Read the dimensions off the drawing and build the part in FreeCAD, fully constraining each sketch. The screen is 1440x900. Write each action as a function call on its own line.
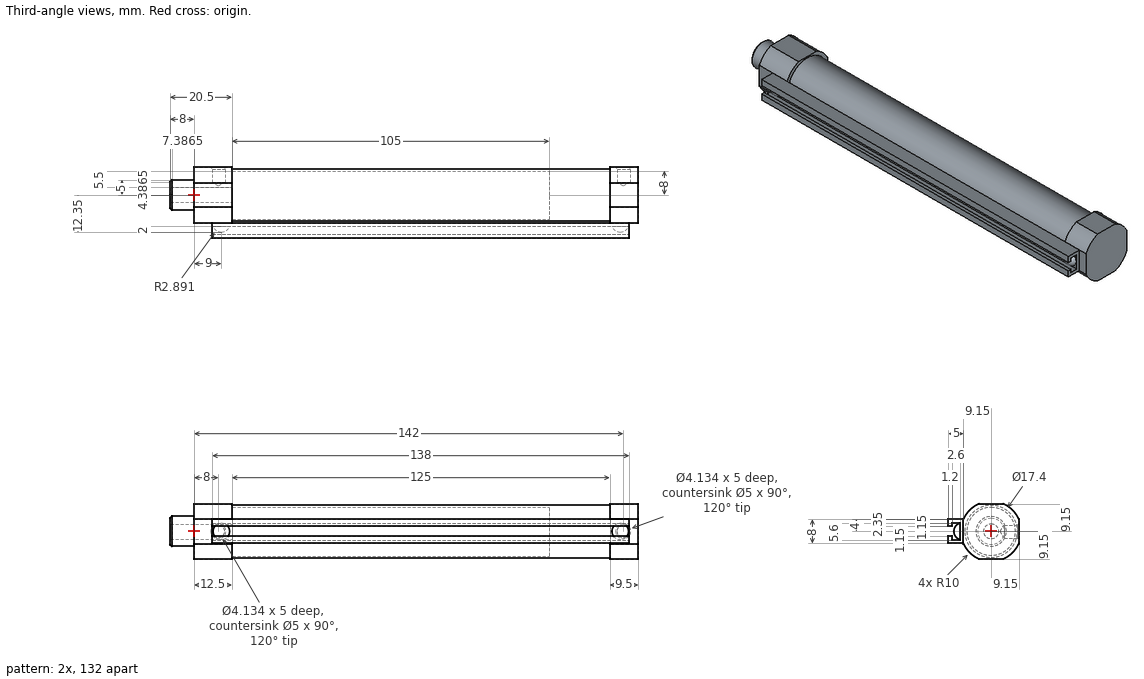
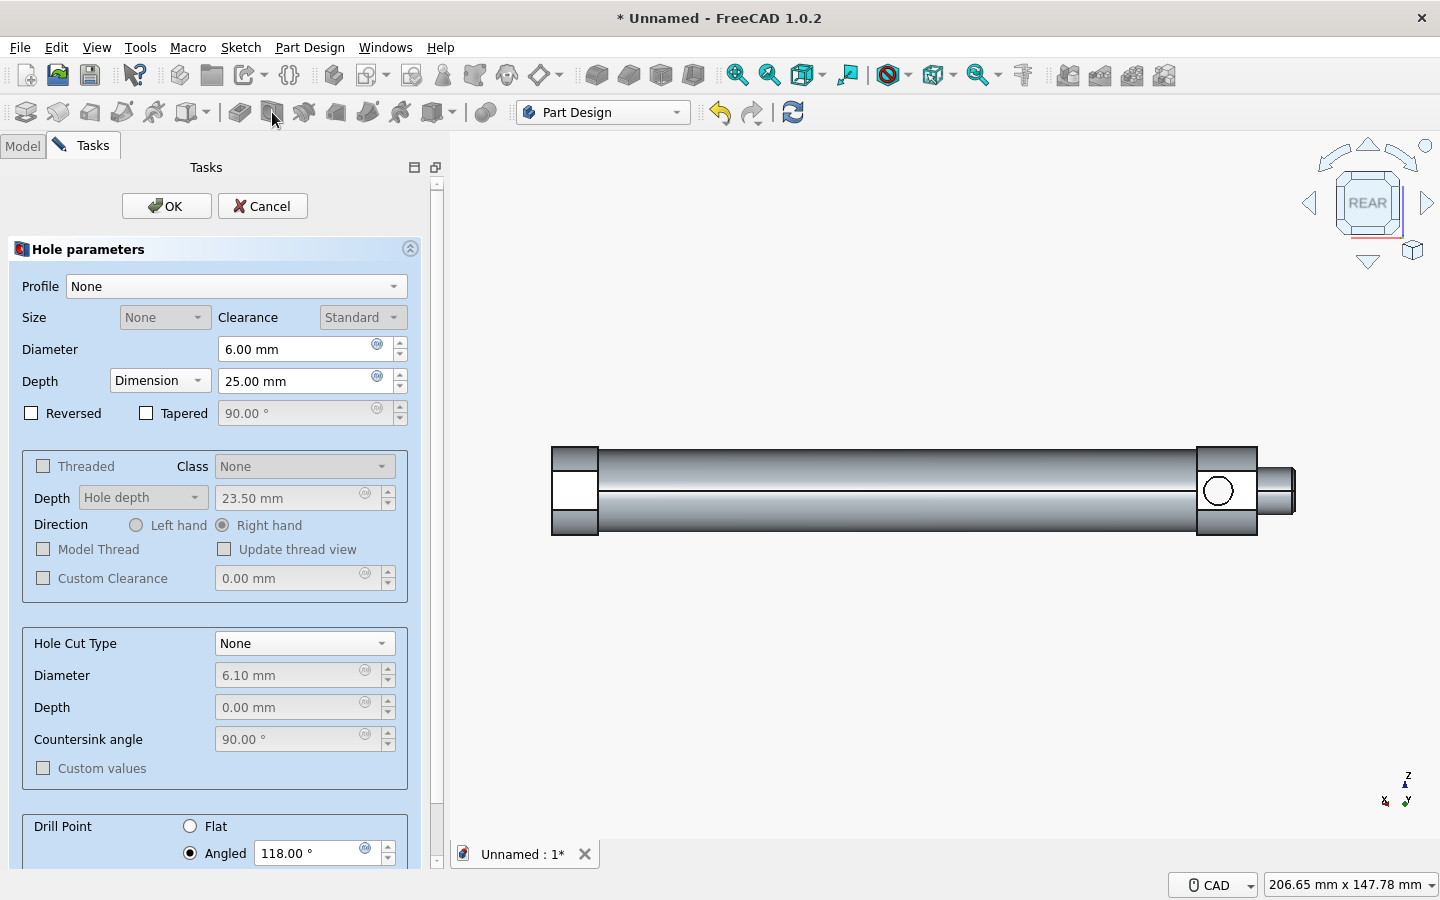
triple_click(305, 349)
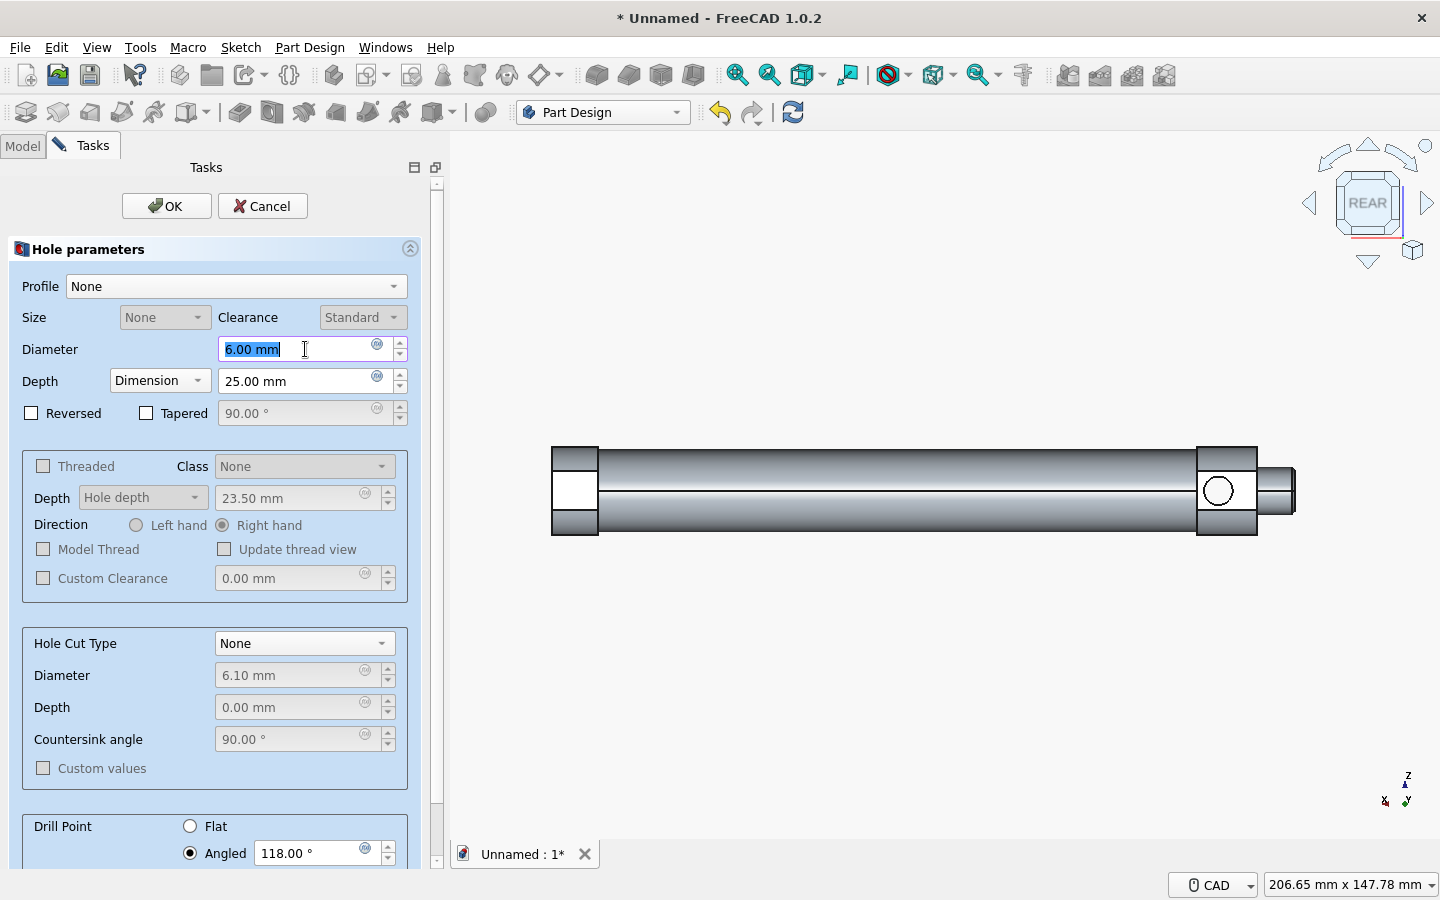
text(4.134)
key(Tab)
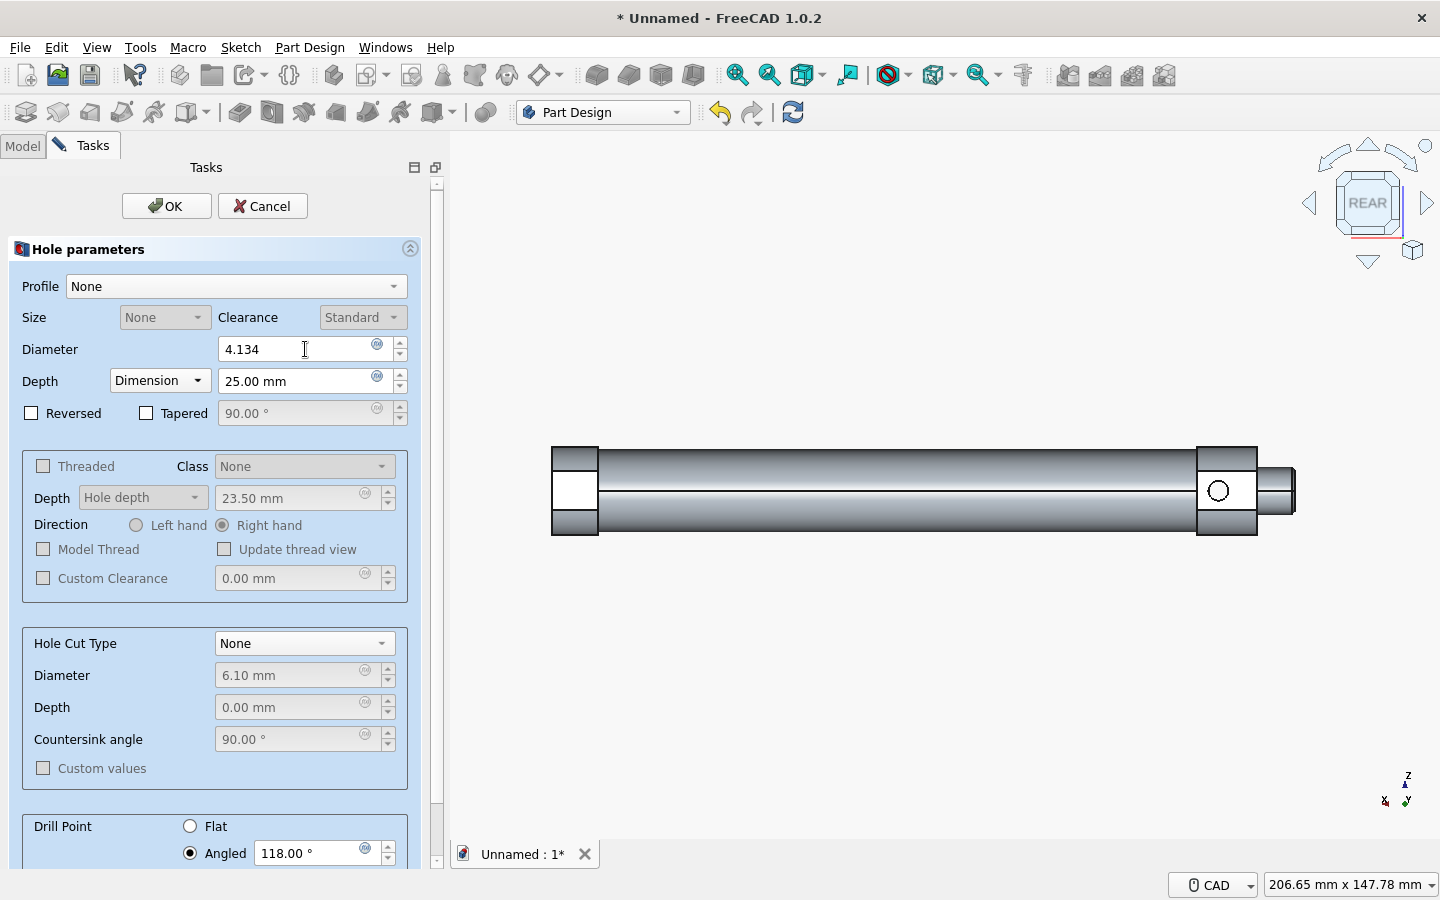
triple_click(305, 381)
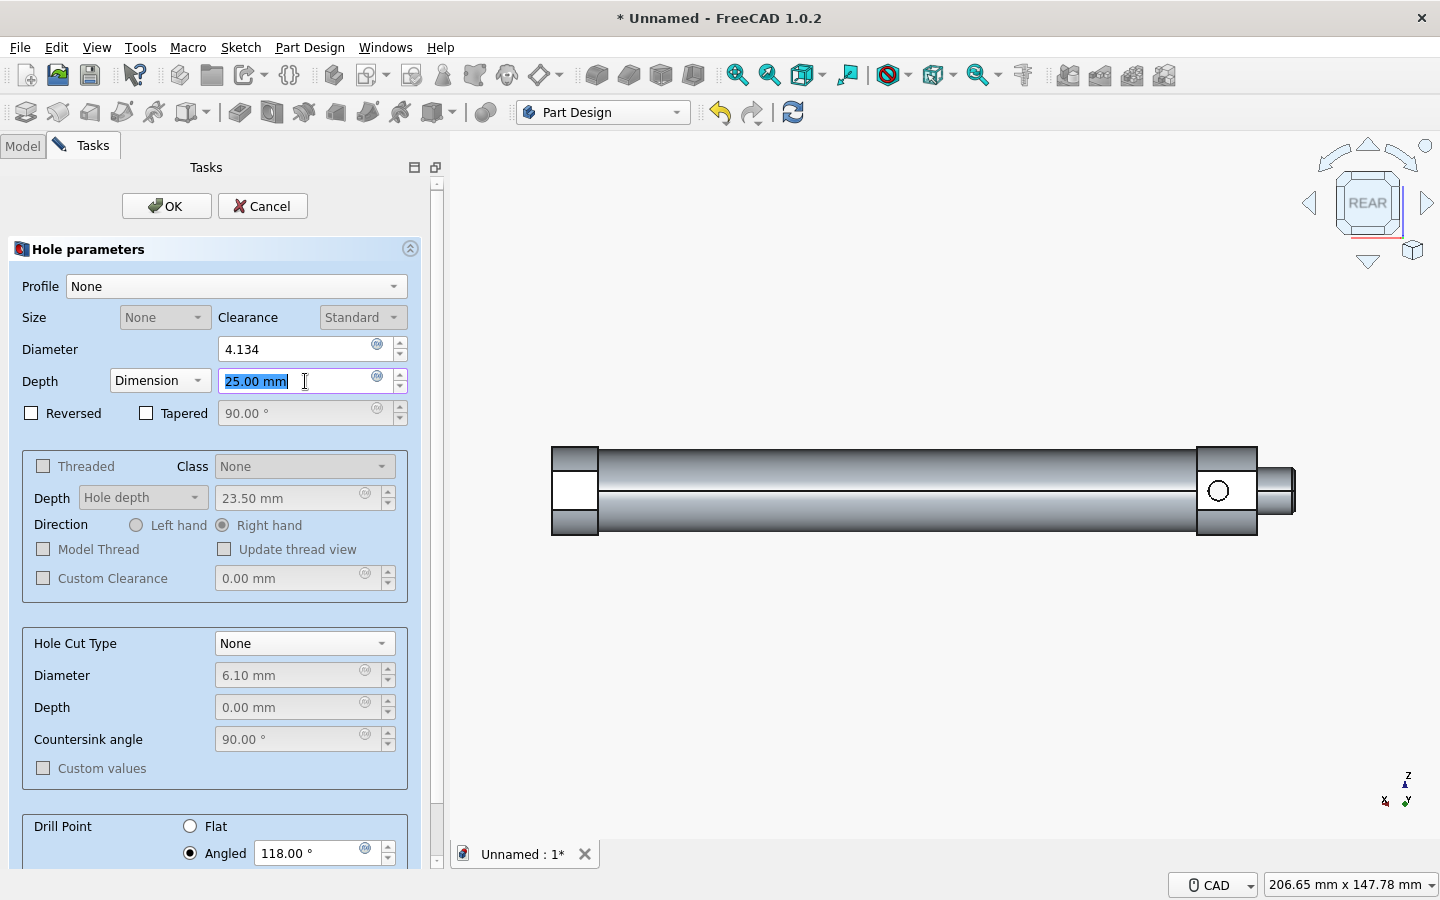
text(5)
key(Tab)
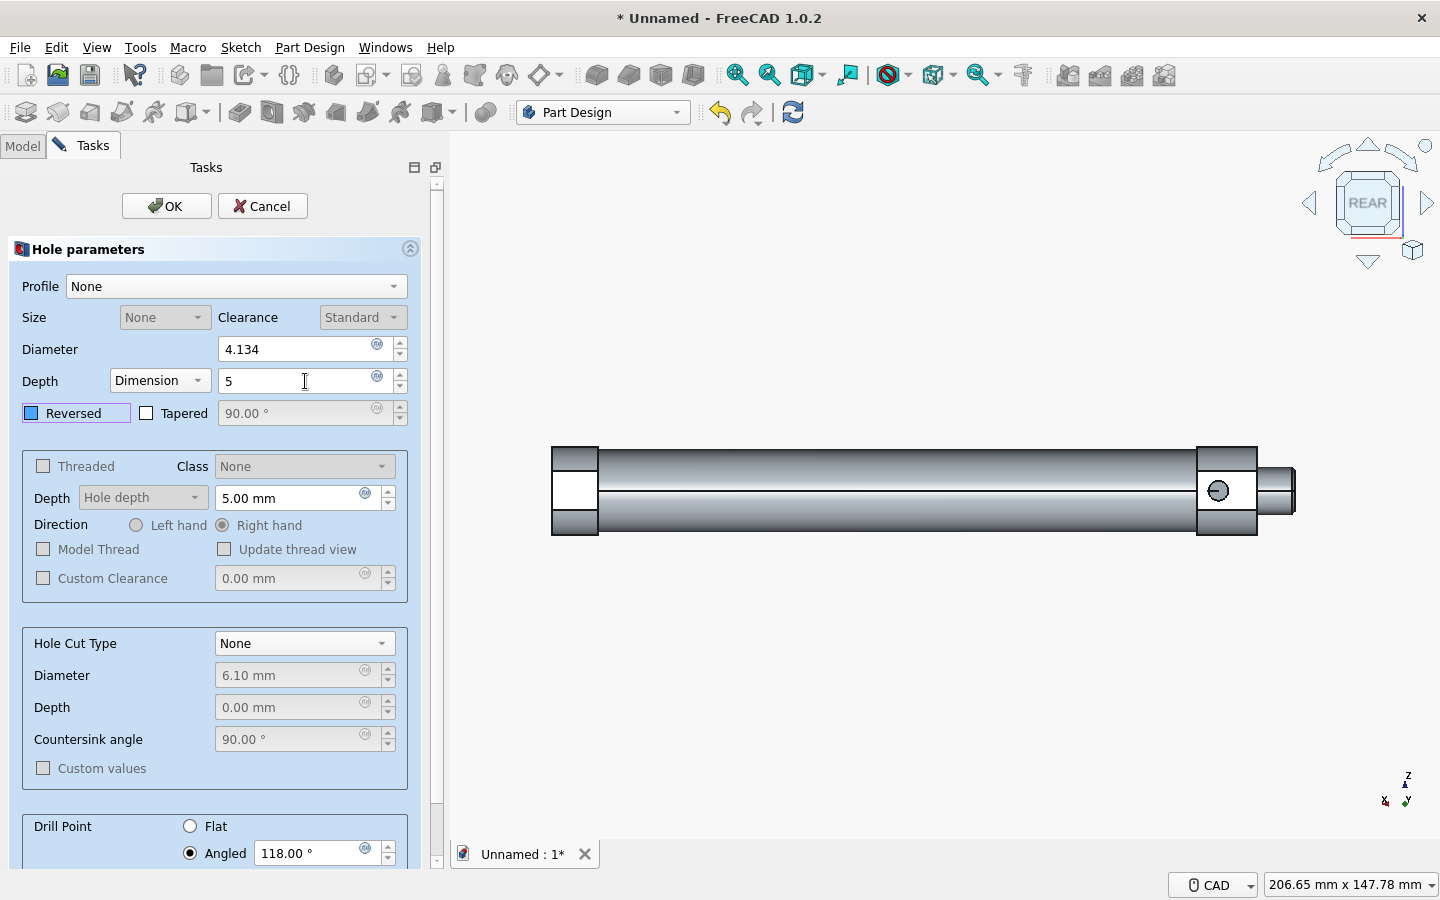
click(306, 644)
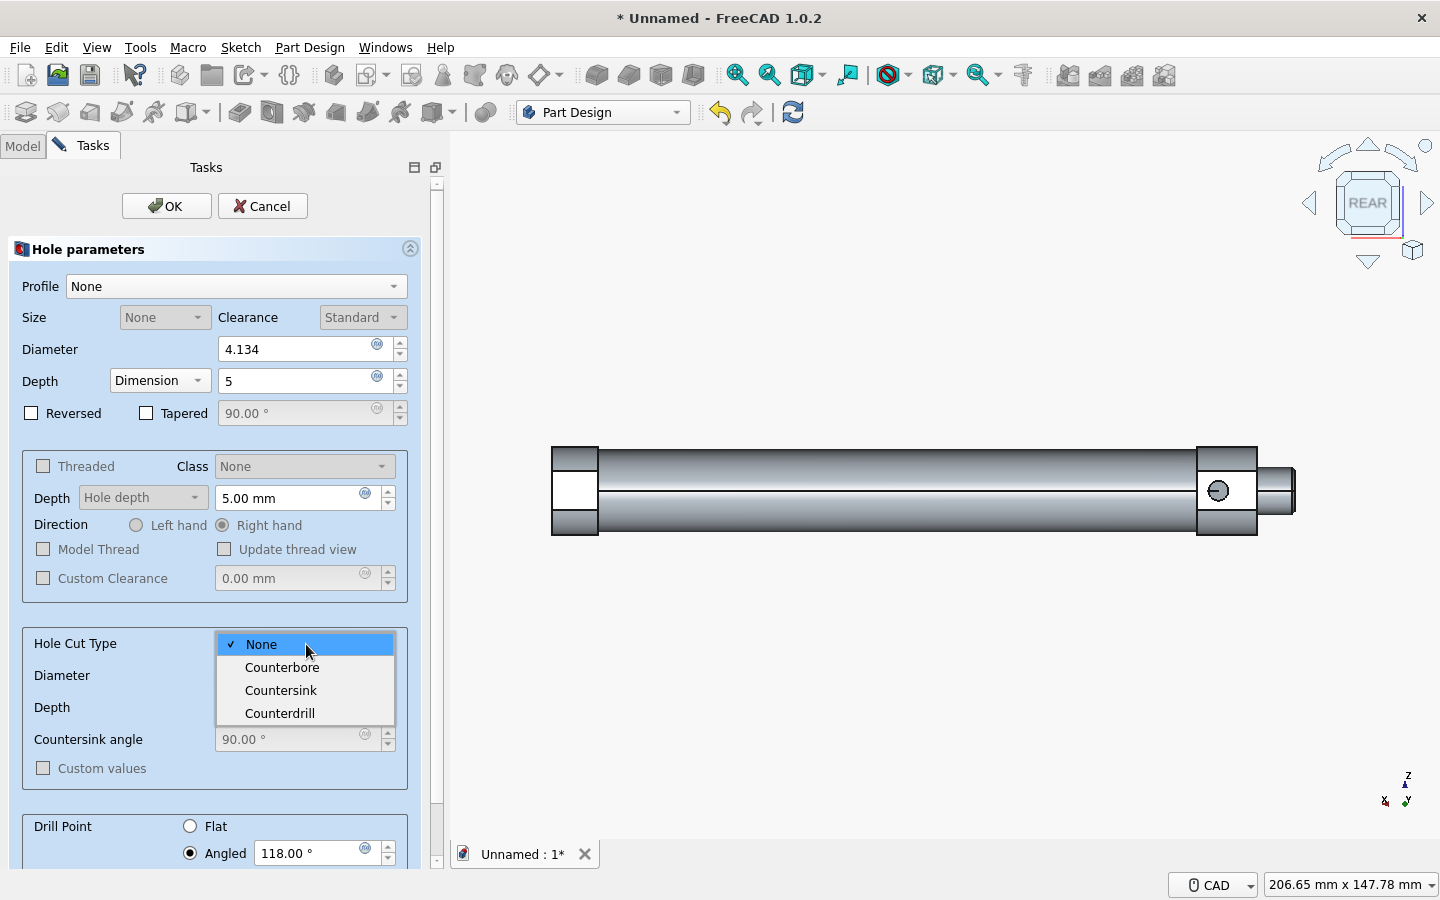
click(304, 690)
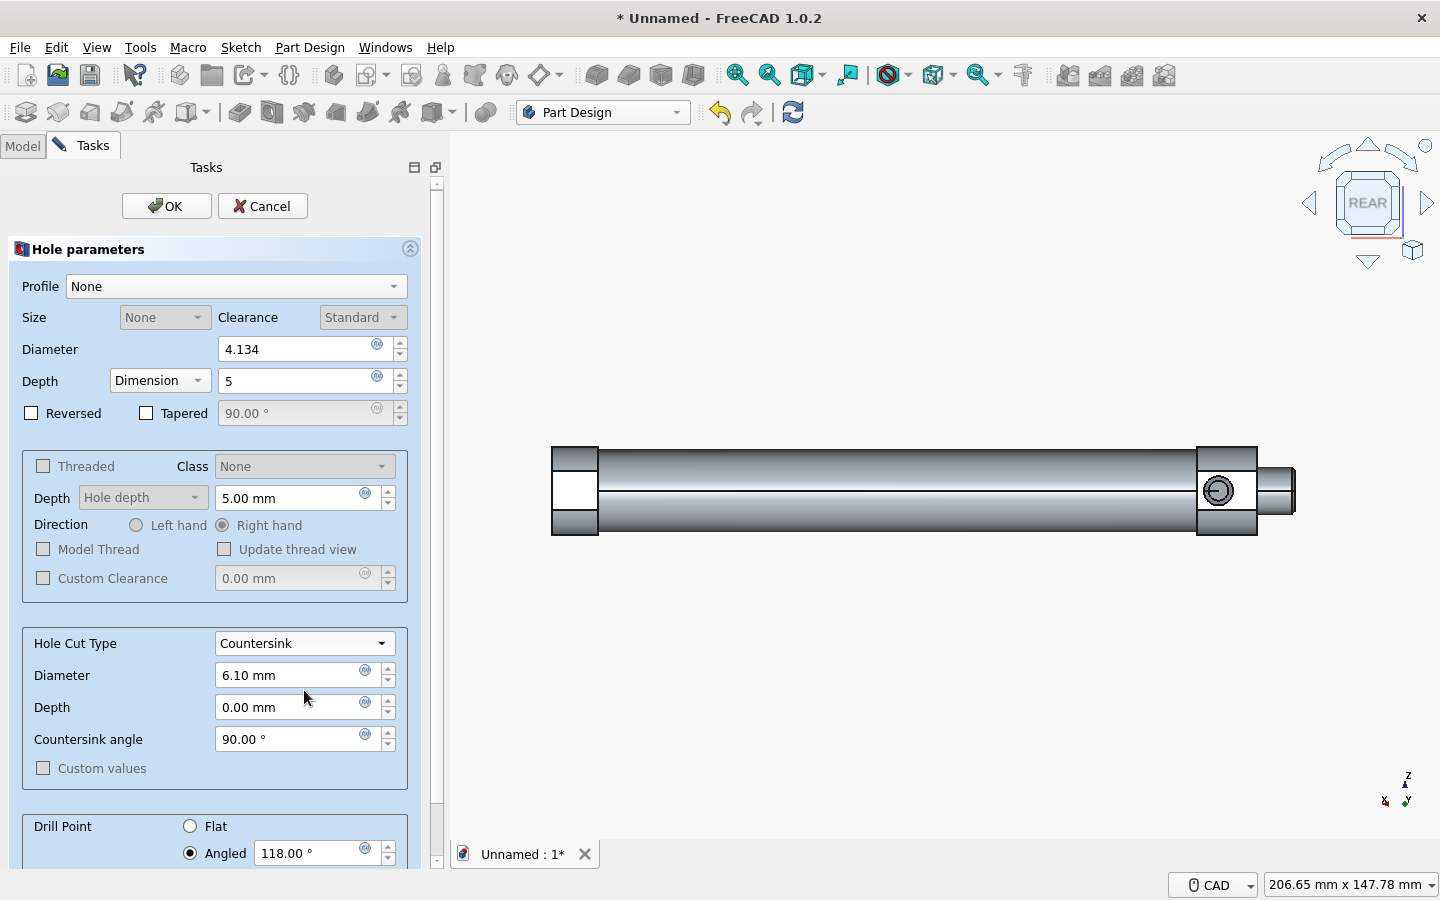
triple_click(298, 675)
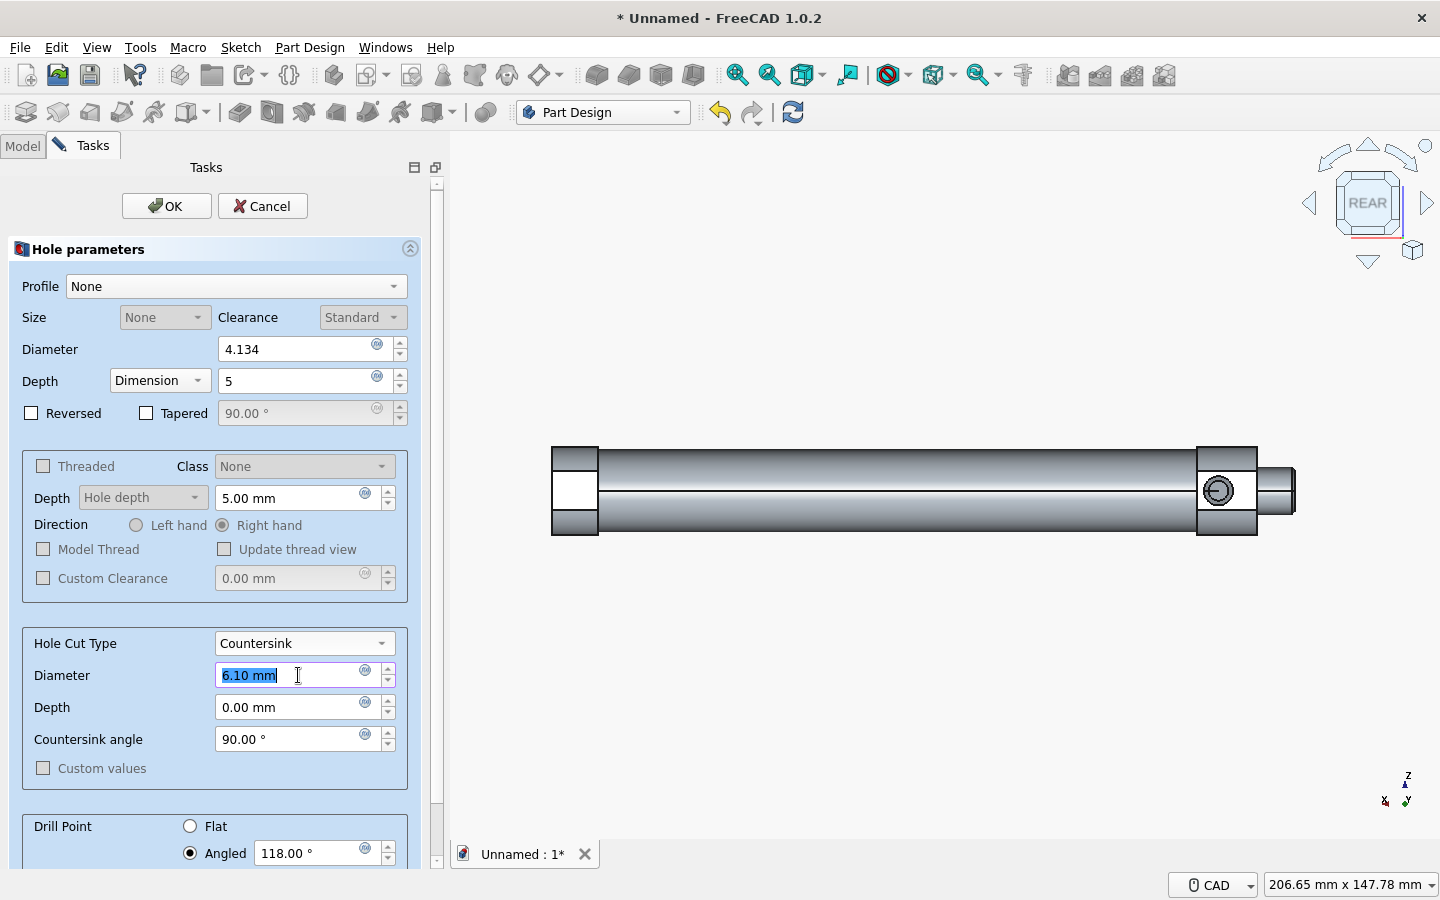
text(5)
key(Tab)